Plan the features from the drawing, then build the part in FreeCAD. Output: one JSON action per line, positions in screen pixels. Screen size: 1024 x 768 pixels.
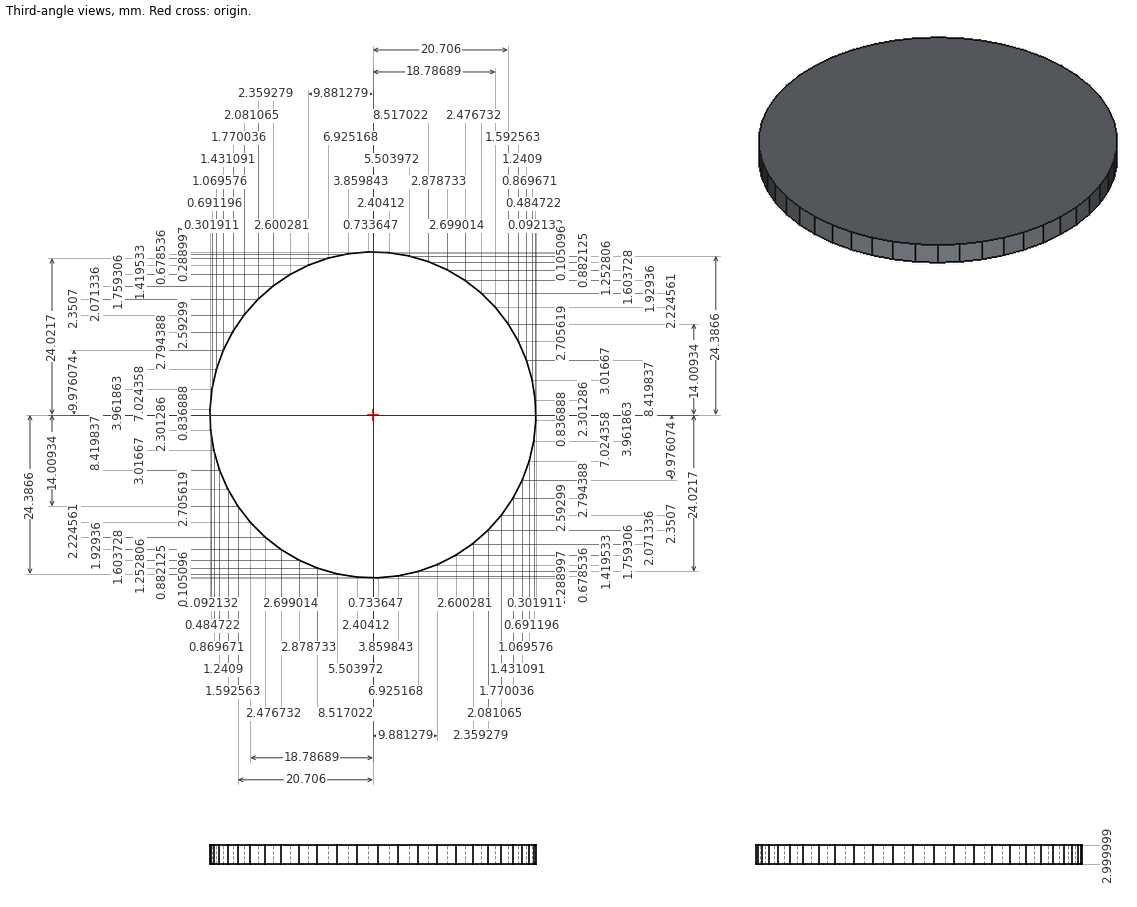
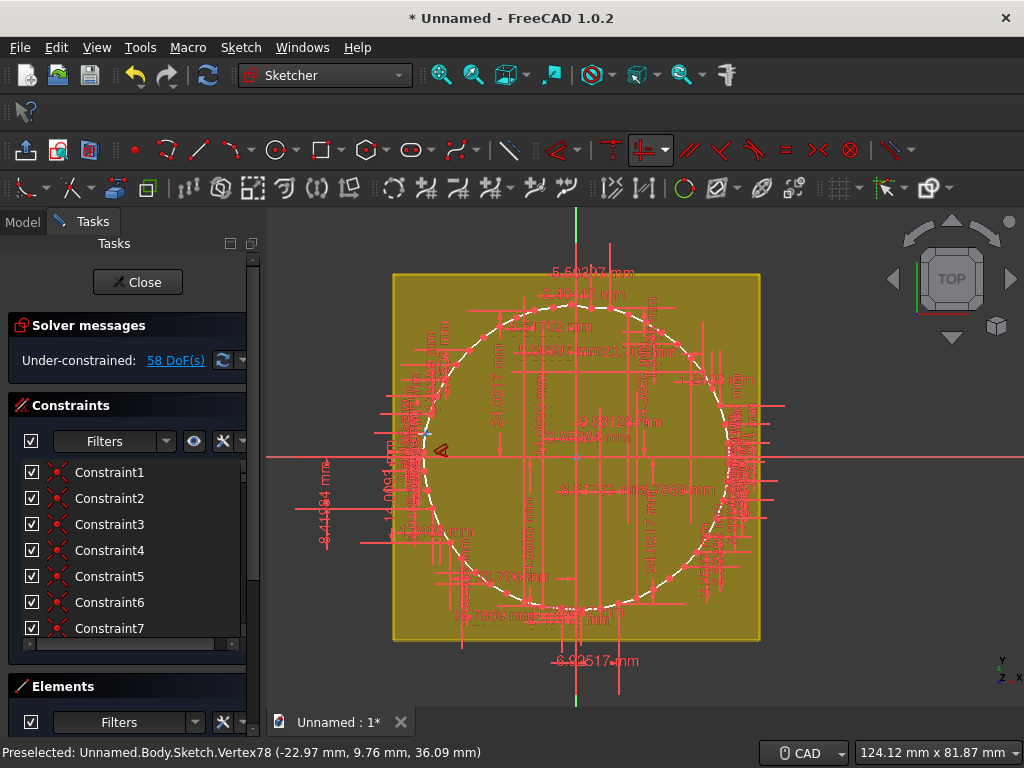
{"action": "left_click", "coordinate": [516, 318]}
{"action": "left_click", "coordinate": [532, 491]}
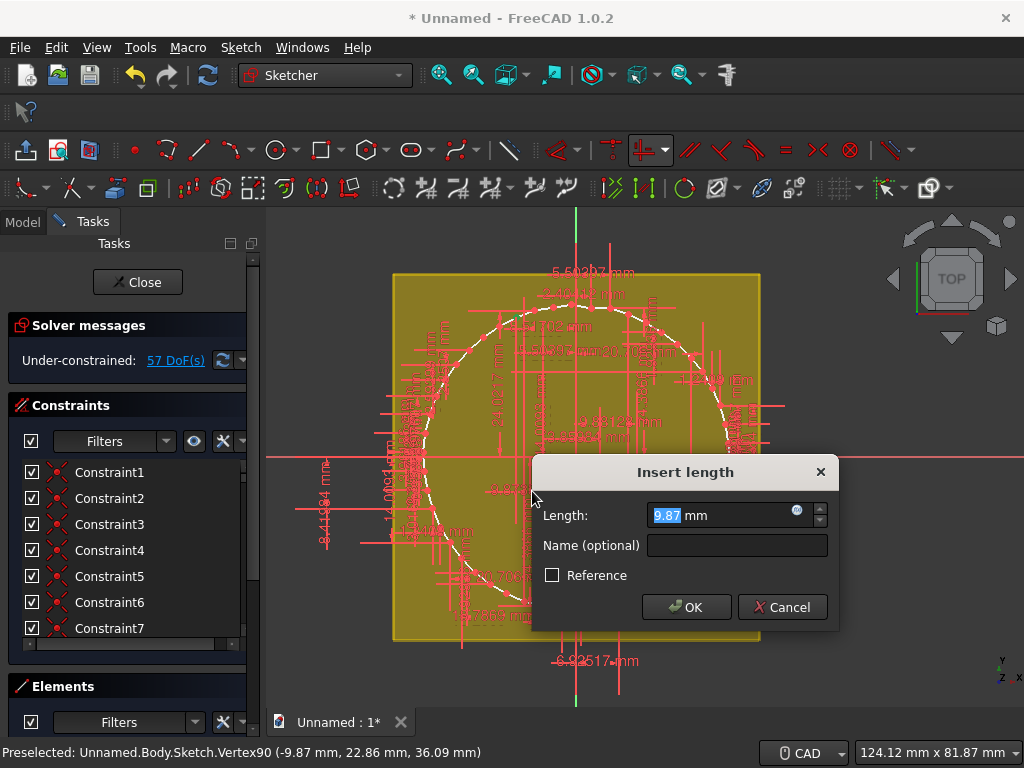
{"action": "type", "text": "9.881279"}
{"action": "key", "text": "Return"}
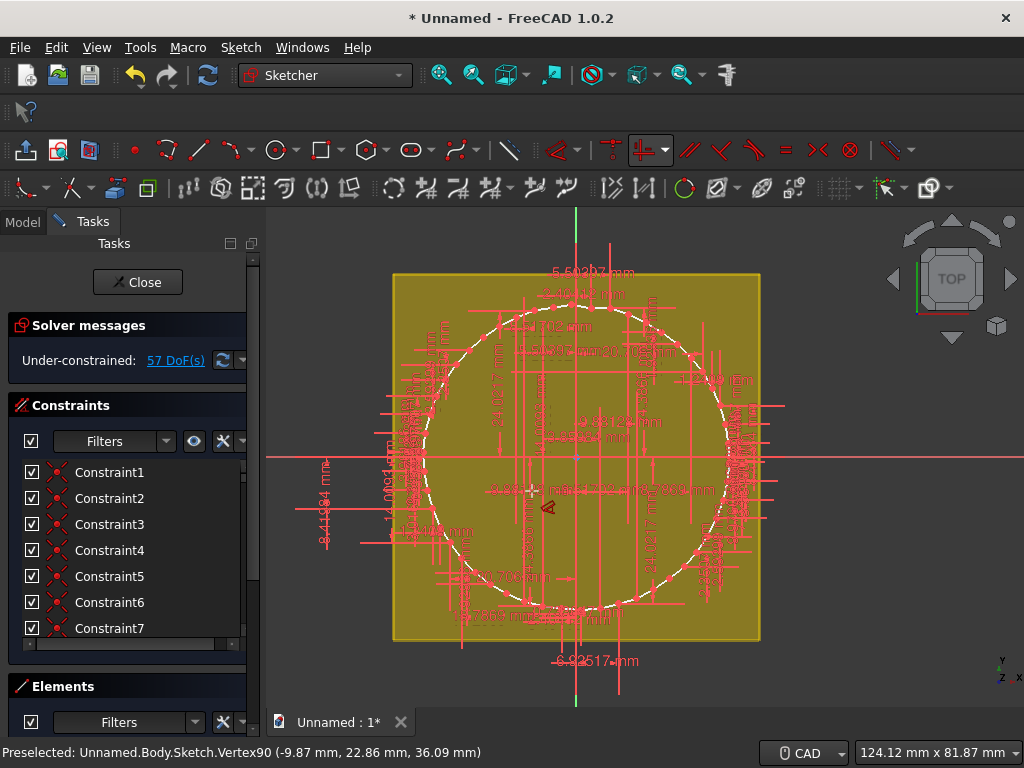
{"action": "left_click", "coordinate": [534, 311]}
{"action": "left_click", "coordinate": [555, 253]}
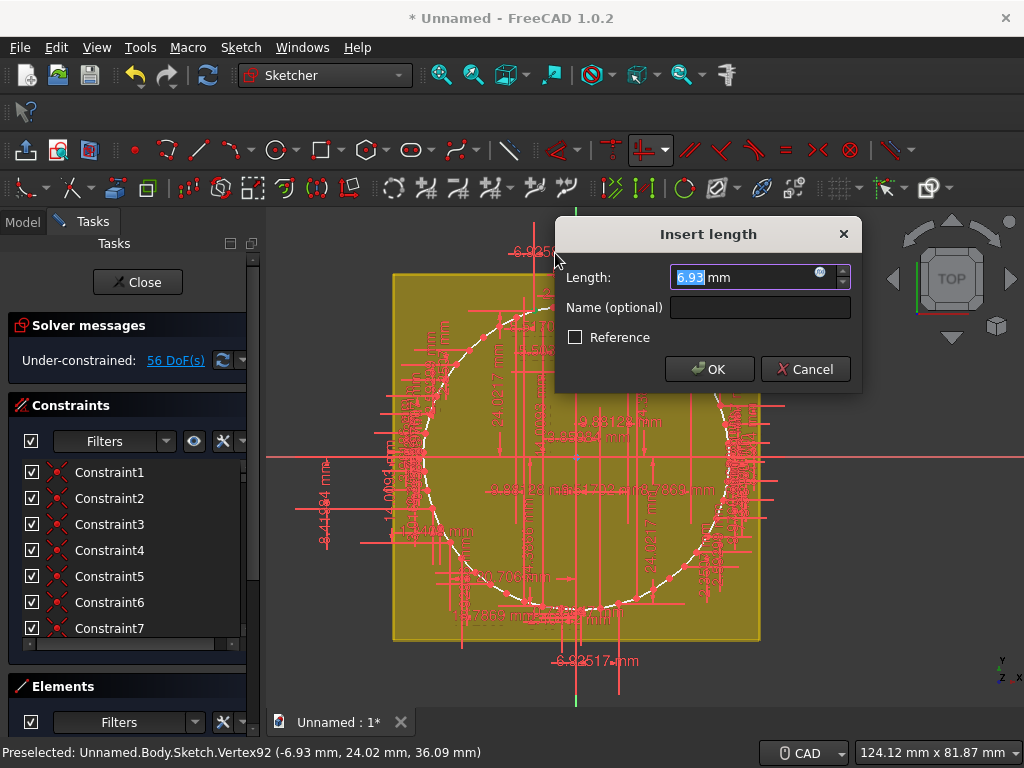
{"action": "type", "text": "6.925168"}
{"action": "key", "text": "Return"}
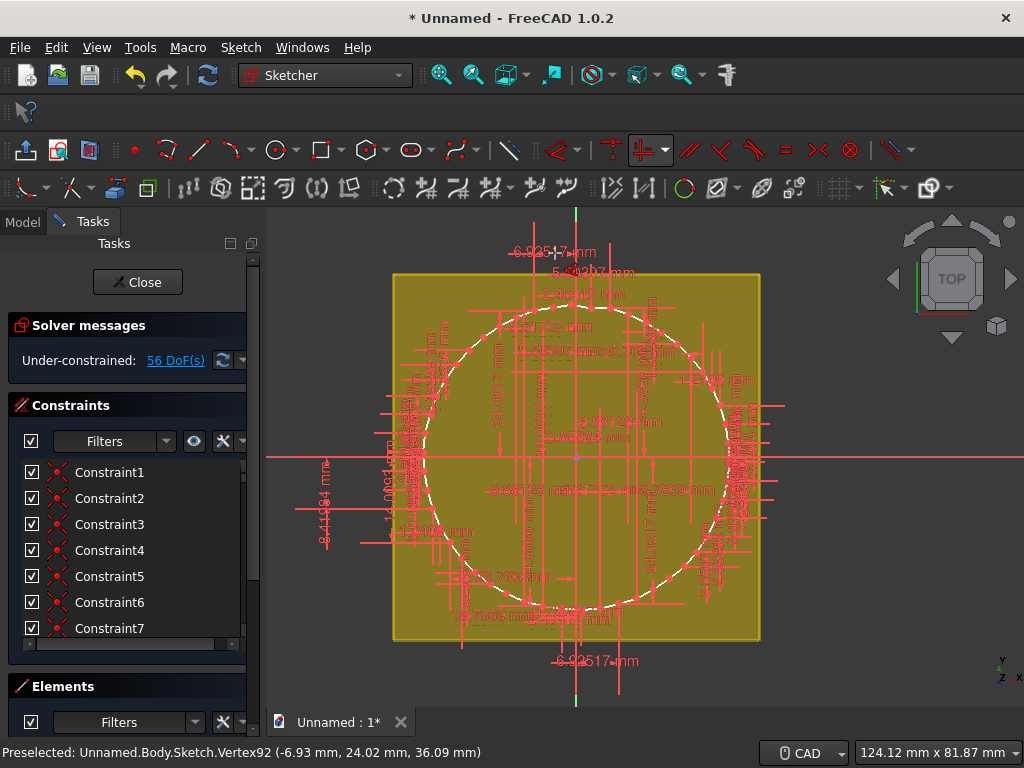
{"action": "scroll", "coordinate": [553, 308], "scroll_direction": "up", "scroll_amount": 3}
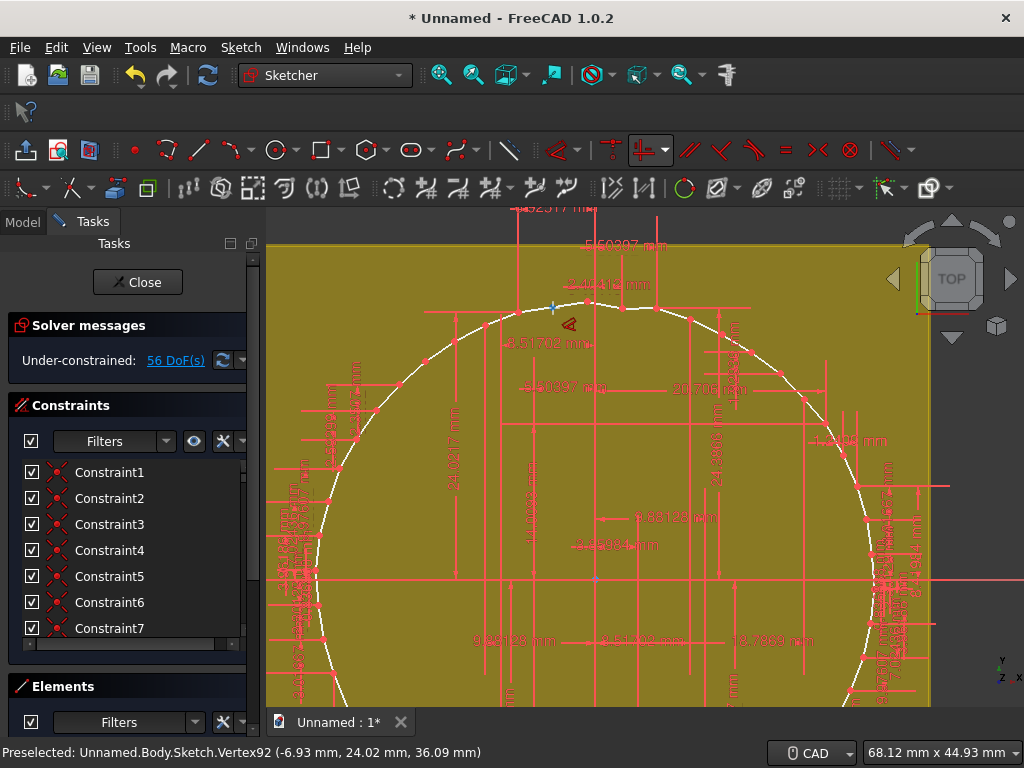
{"action": "left_click", "coordinate": [553, 307]}
{"action": "left_click", "coordinate": [574, 614]}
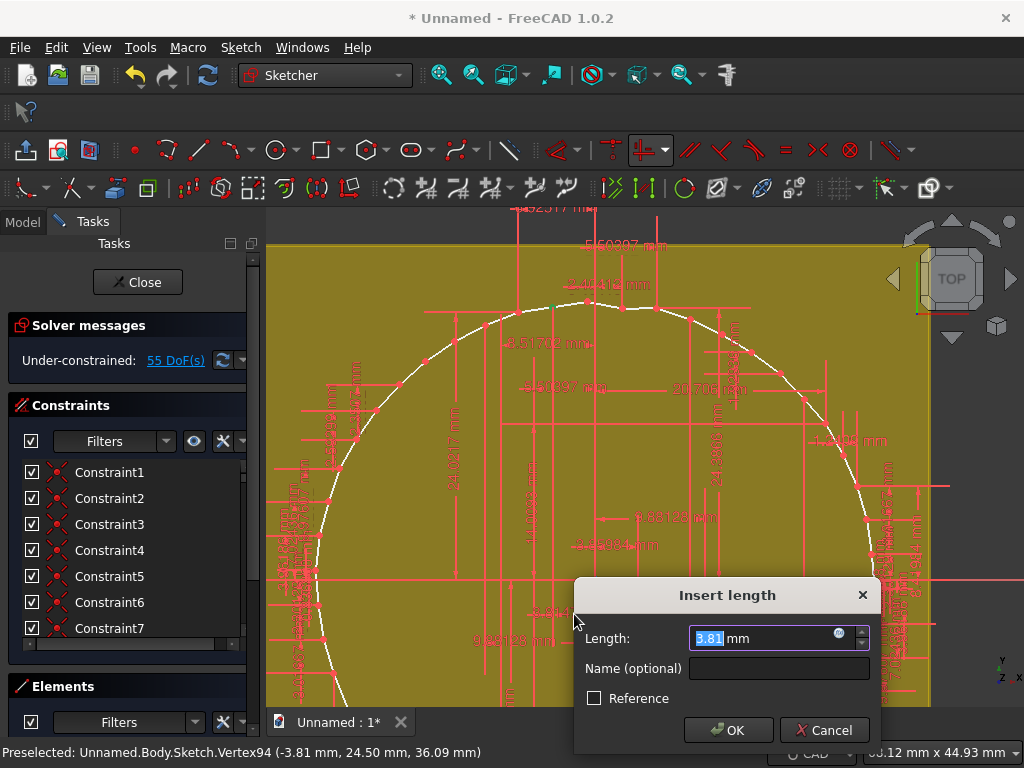
{"action": "type", "text": "3.859843"}
{"action": "key", "text": "Return"}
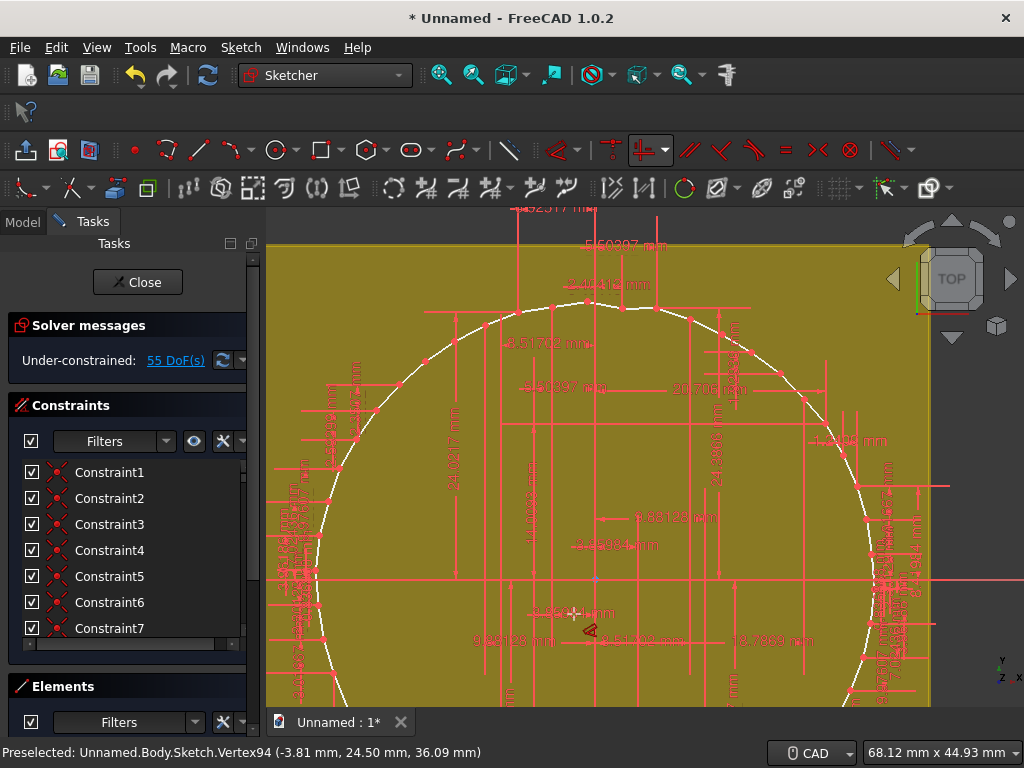
{"action": "scroll", "coordinate": [587, 302], "scroll_direction": "up", "scroll_amount": 8}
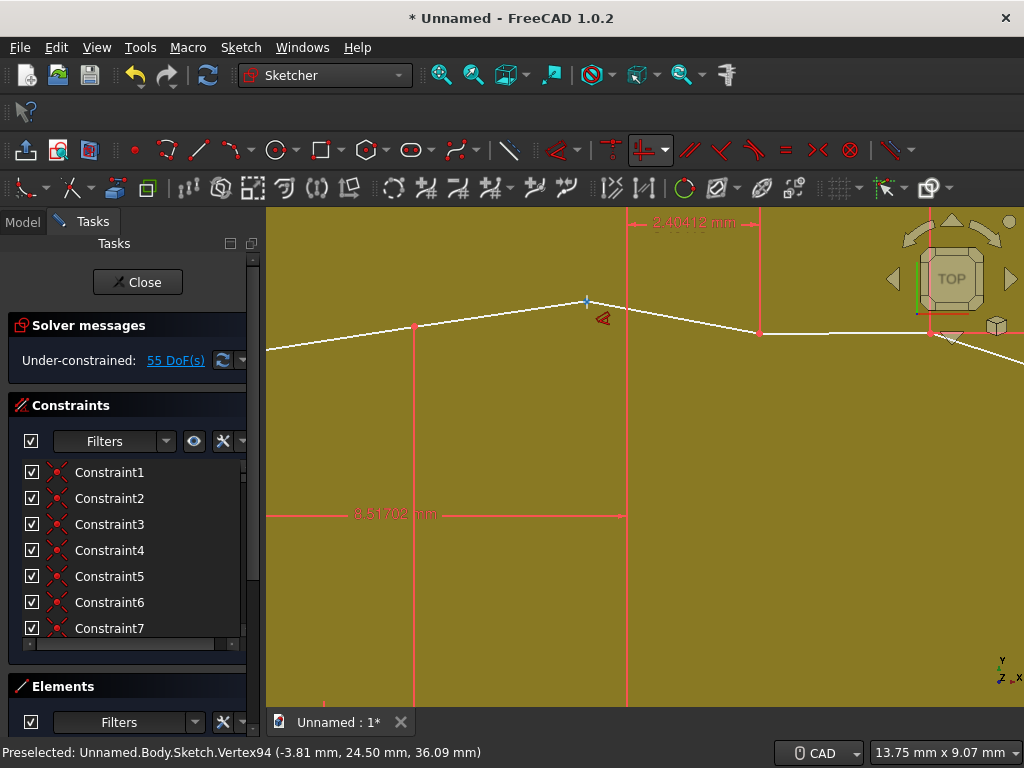
{"action": "left_click", "coordinate": [587, 301]}
{"action": "left_click", "coordinate": [607, 267]}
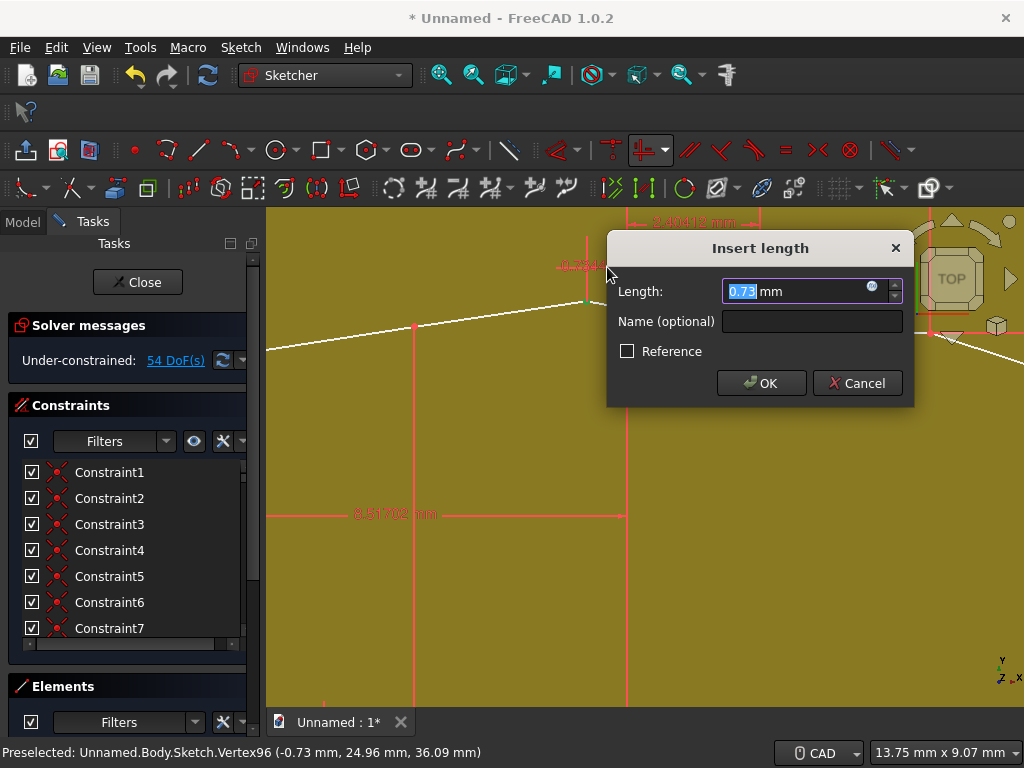
{"action": "type", "text": "0.733647"}
{"action": "key", "text": "Return"}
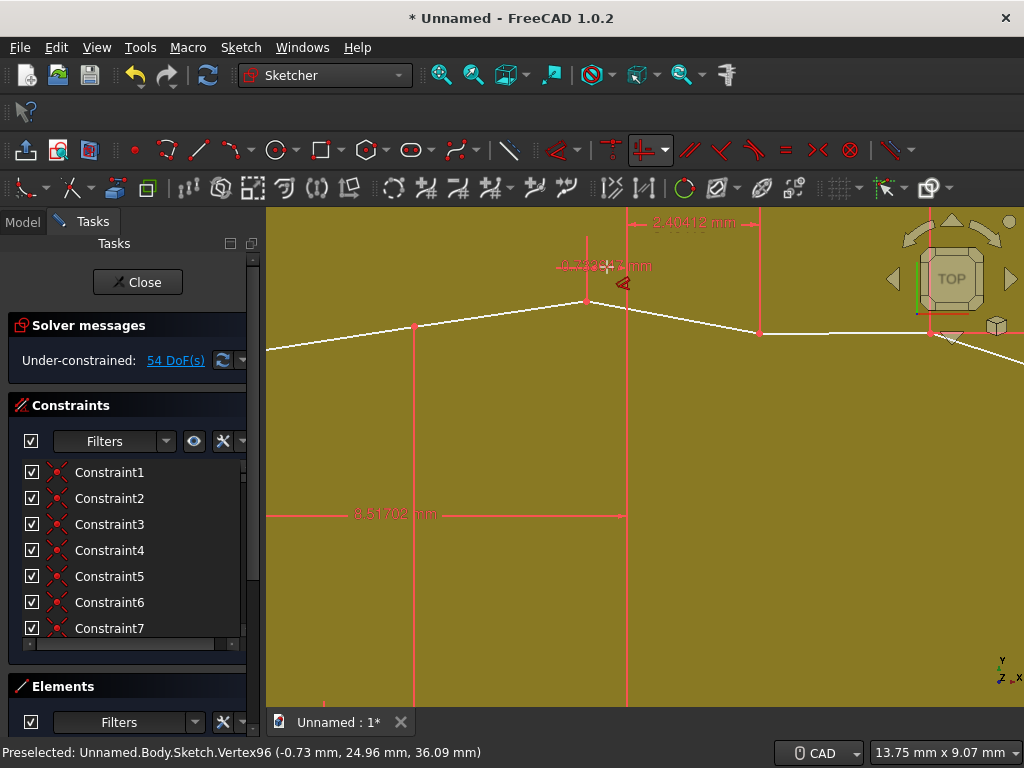
{"action": "scroll", "coordinate": [570, 305], "scroll_direction": "down", "scroll_amount": 11}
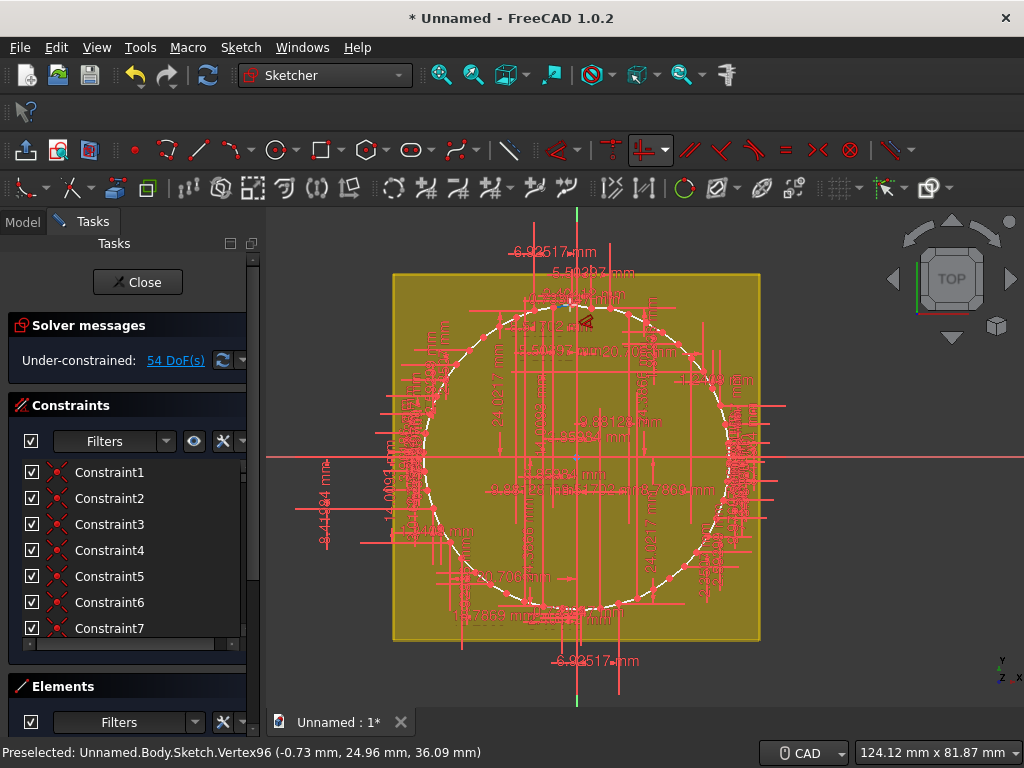
{"action": "scroll", "coordinate": [616, 310], "scroll_direction": "up", "scroll_amount": 10}